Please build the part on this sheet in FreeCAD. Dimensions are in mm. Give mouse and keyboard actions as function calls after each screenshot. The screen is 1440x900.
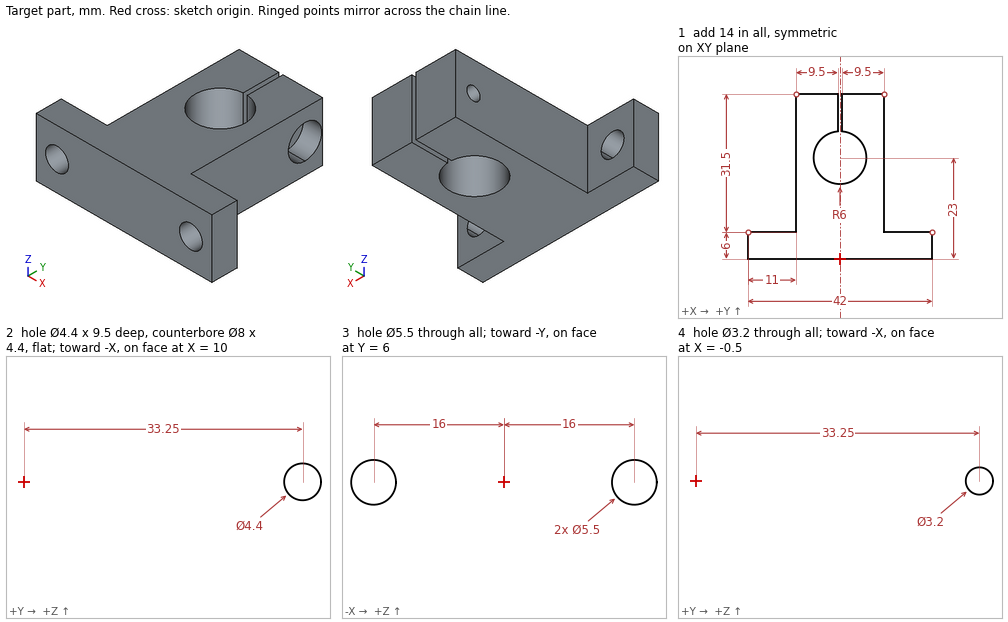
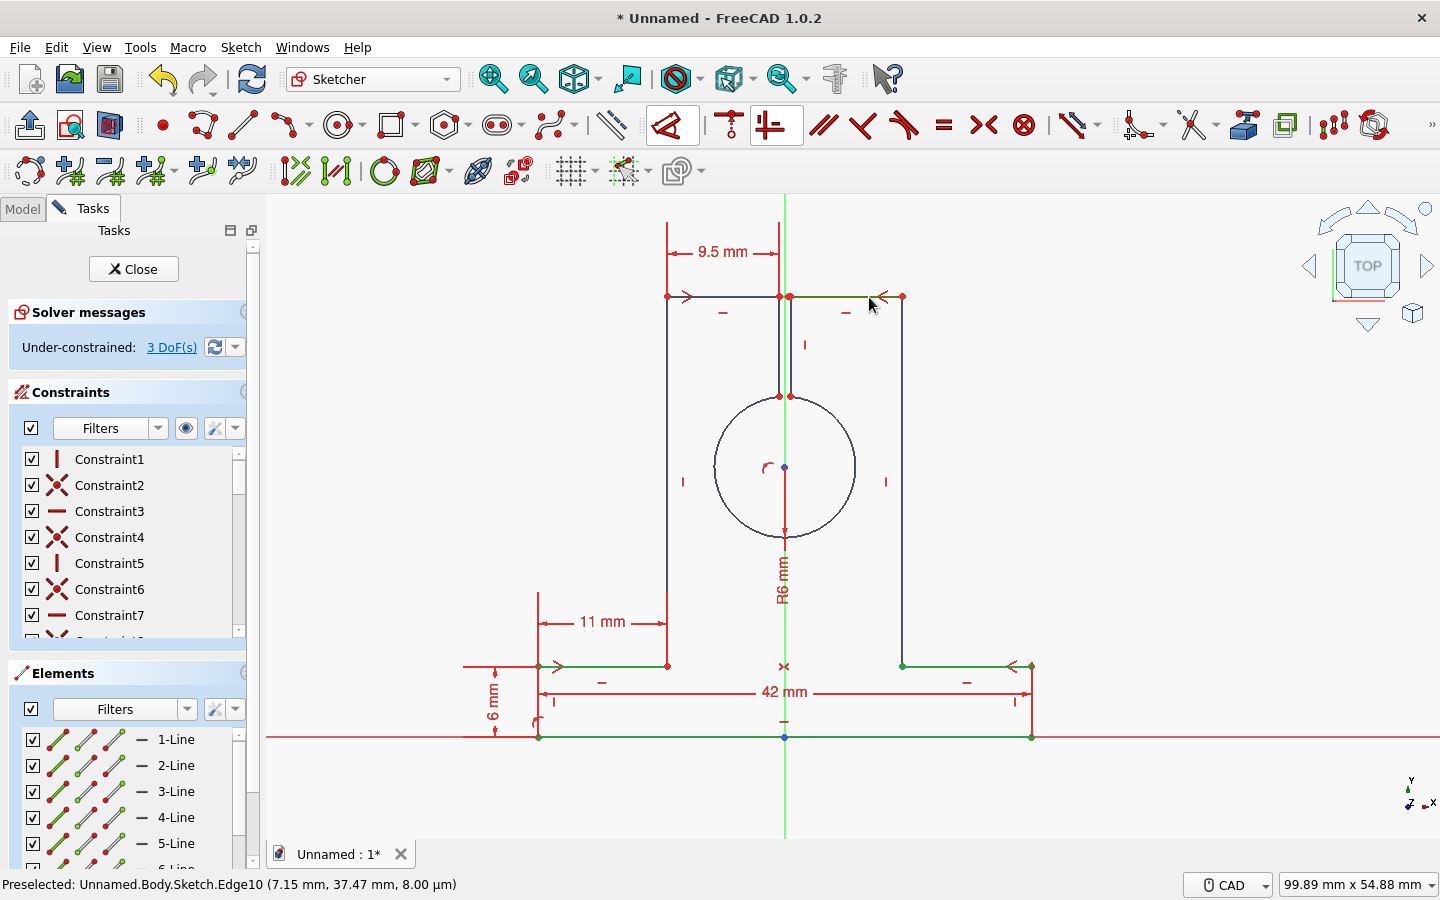
click(694, 126)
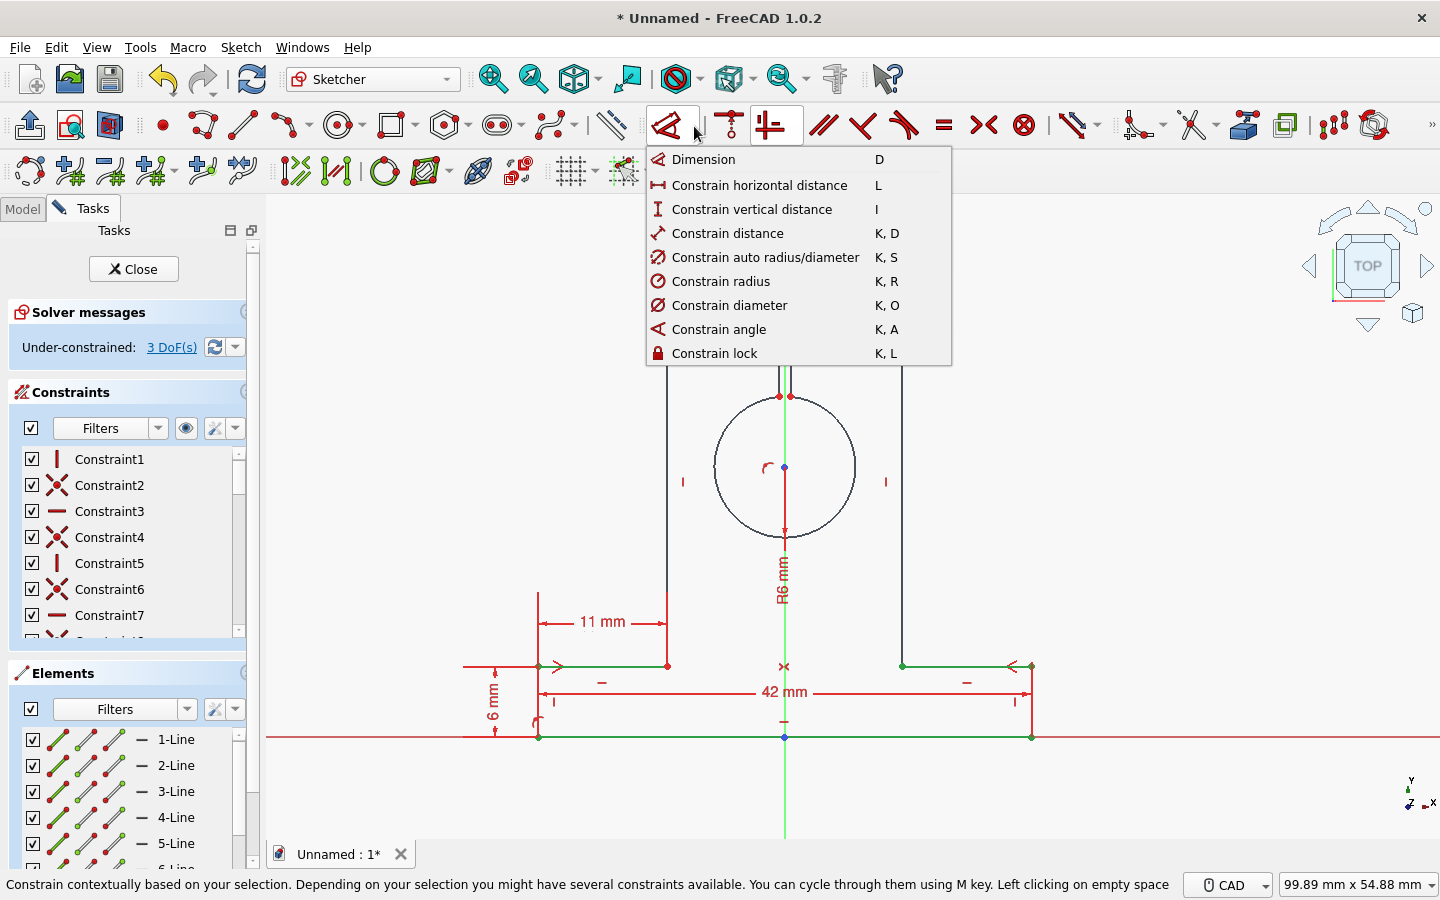
click(799, 185)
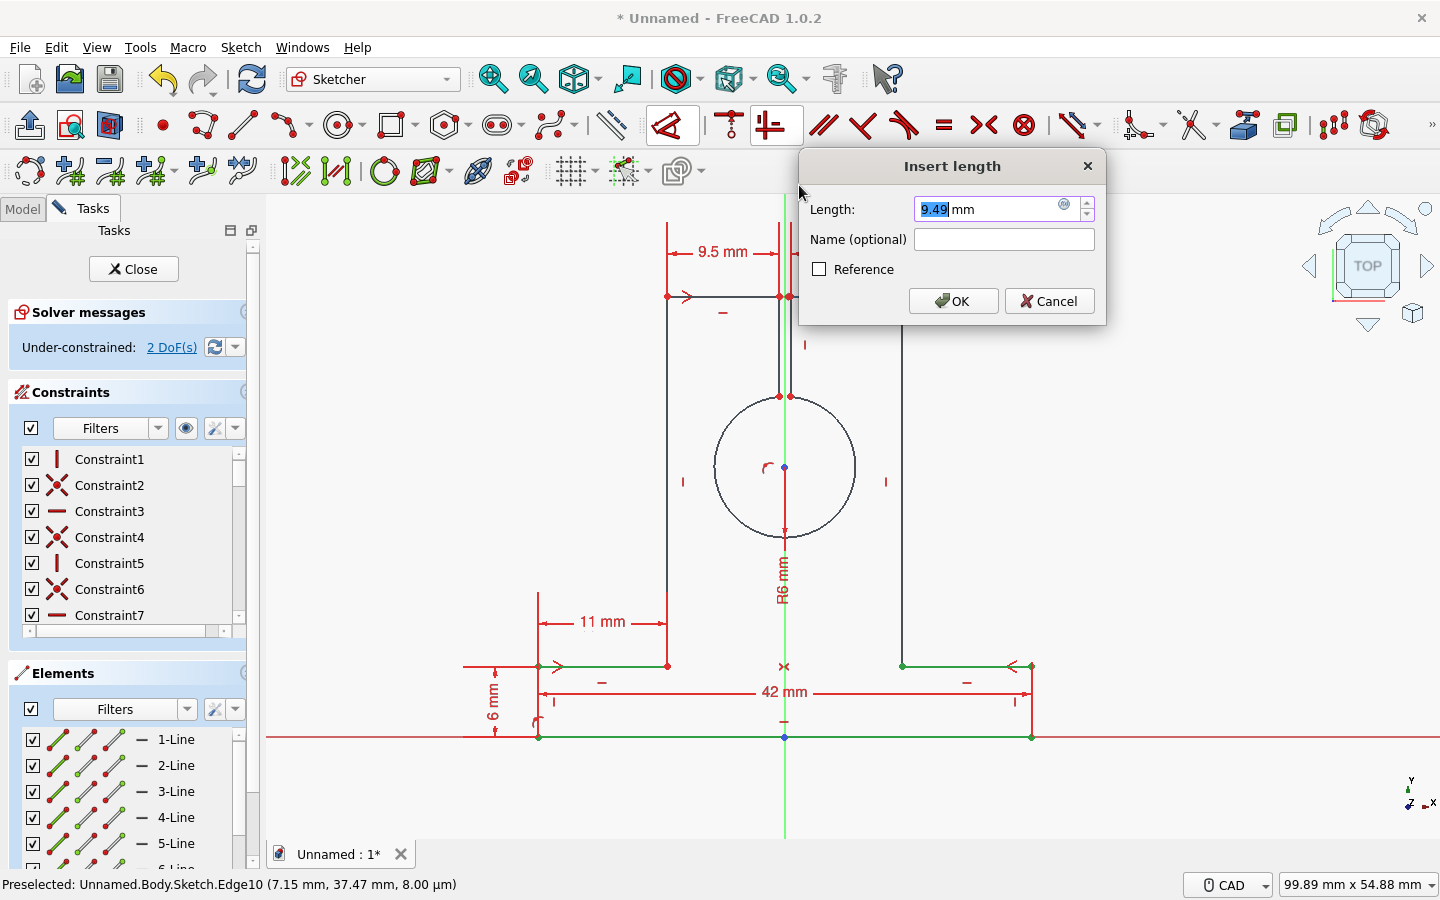
text(9.5)
key(Return)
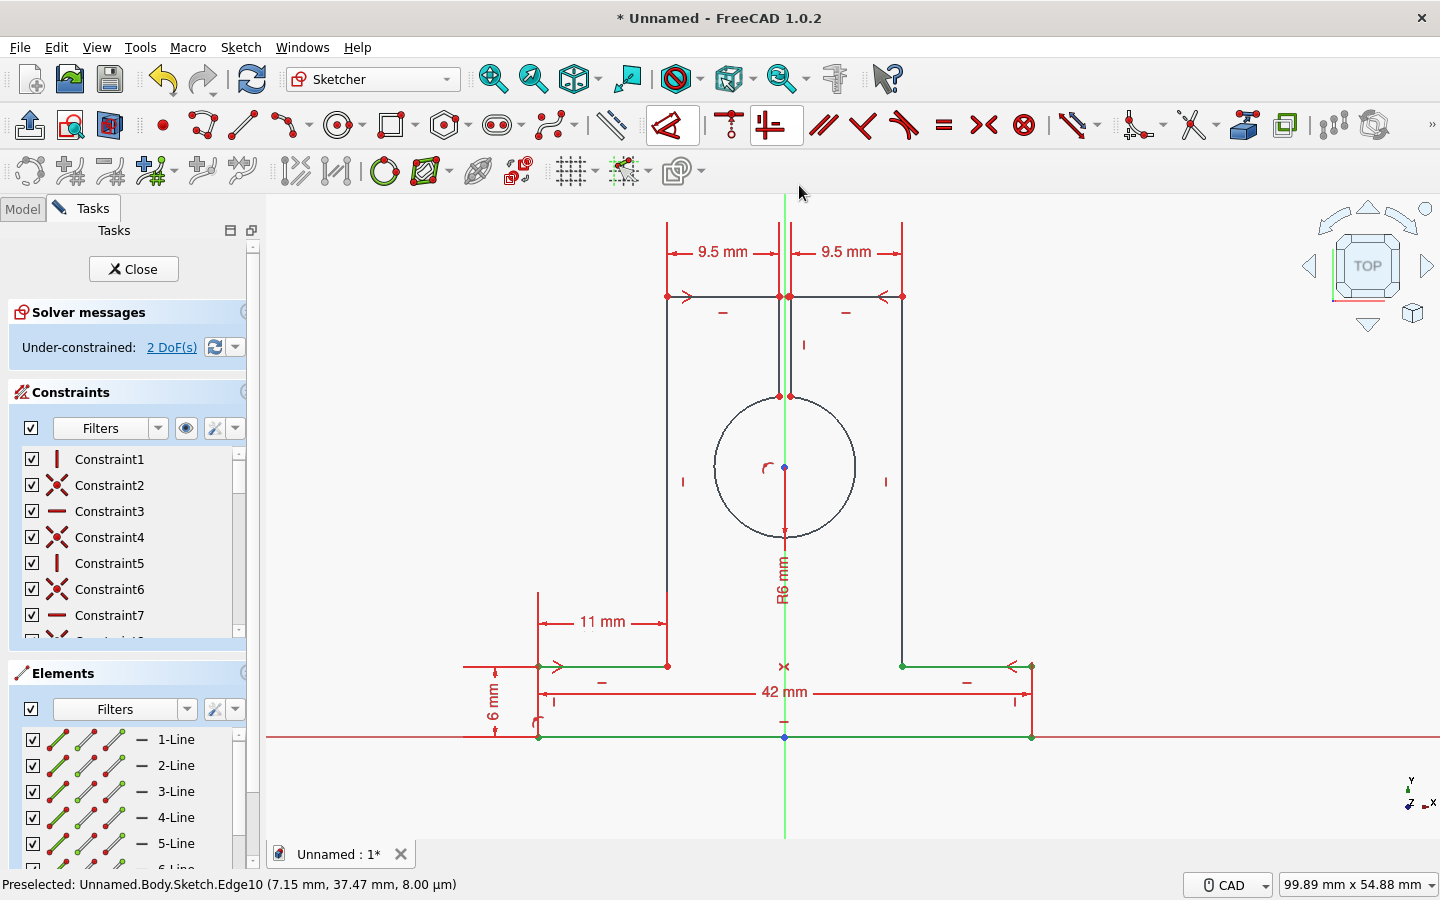
click(785, 467)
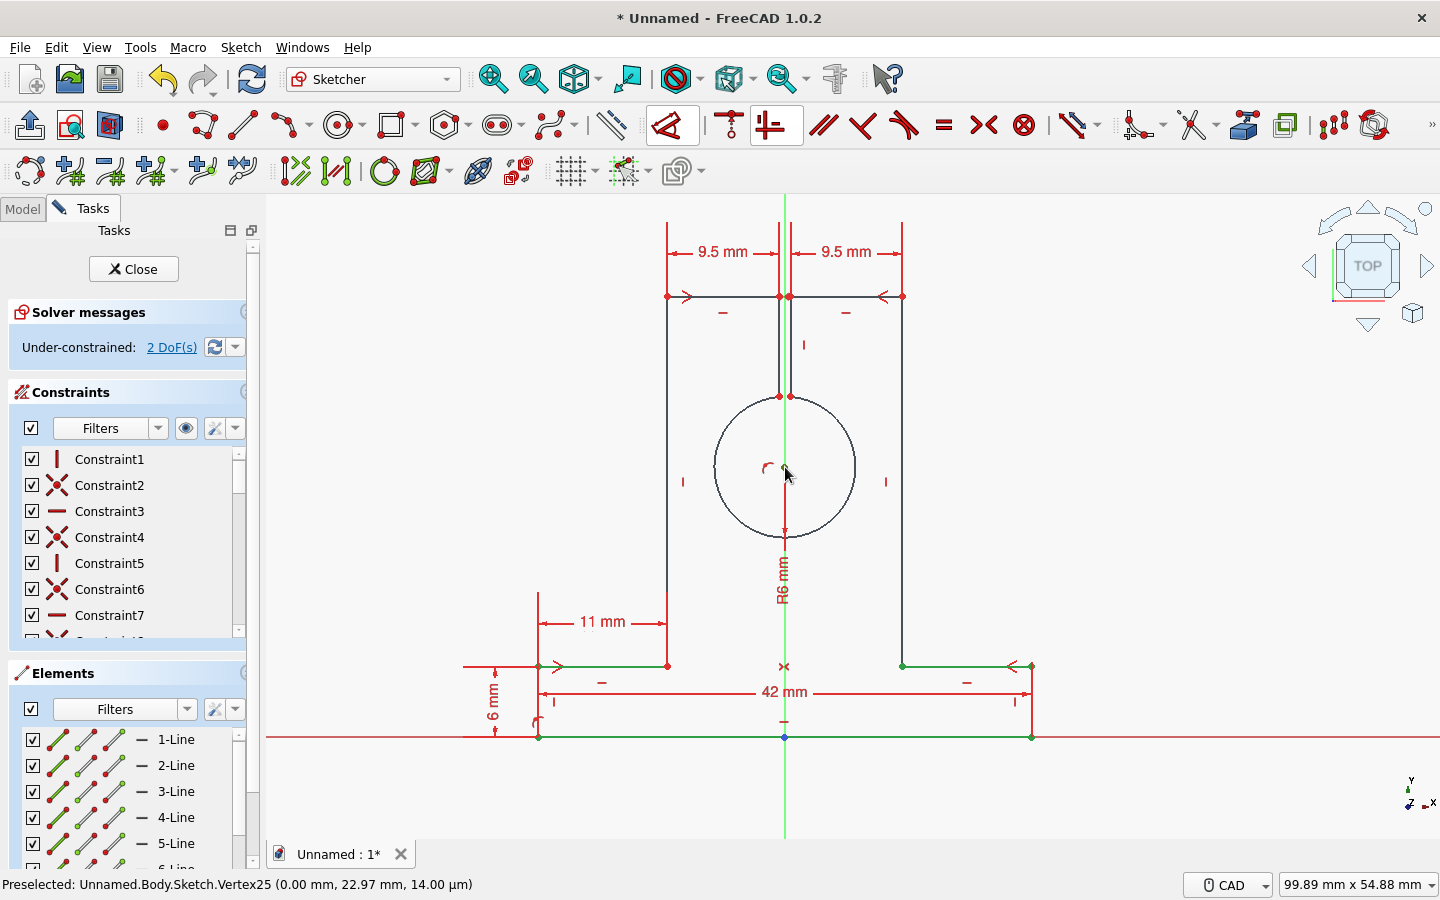
key(i)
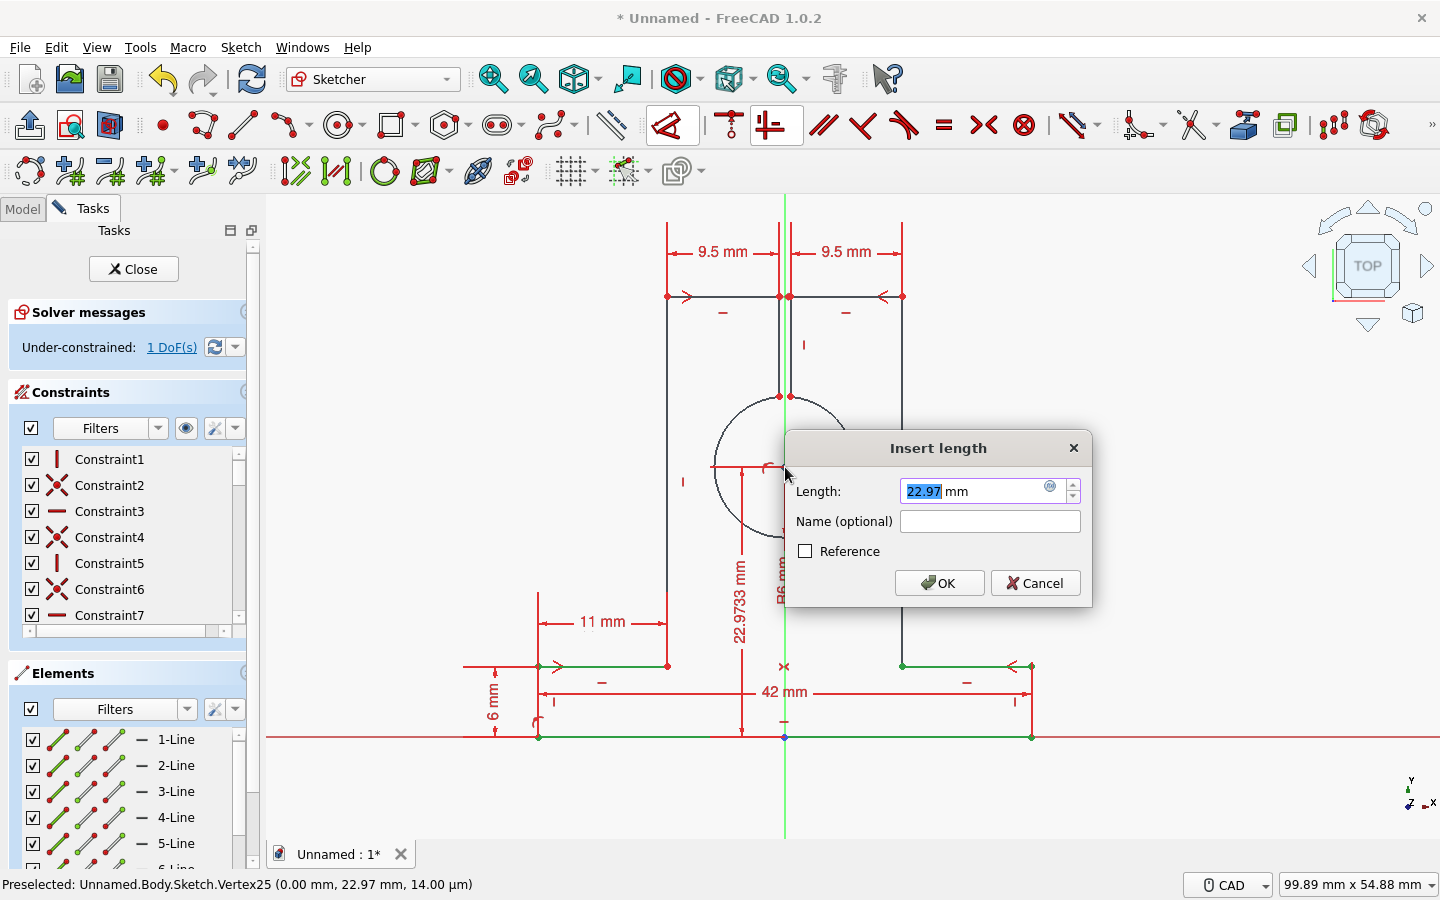
text(23)
key(Return)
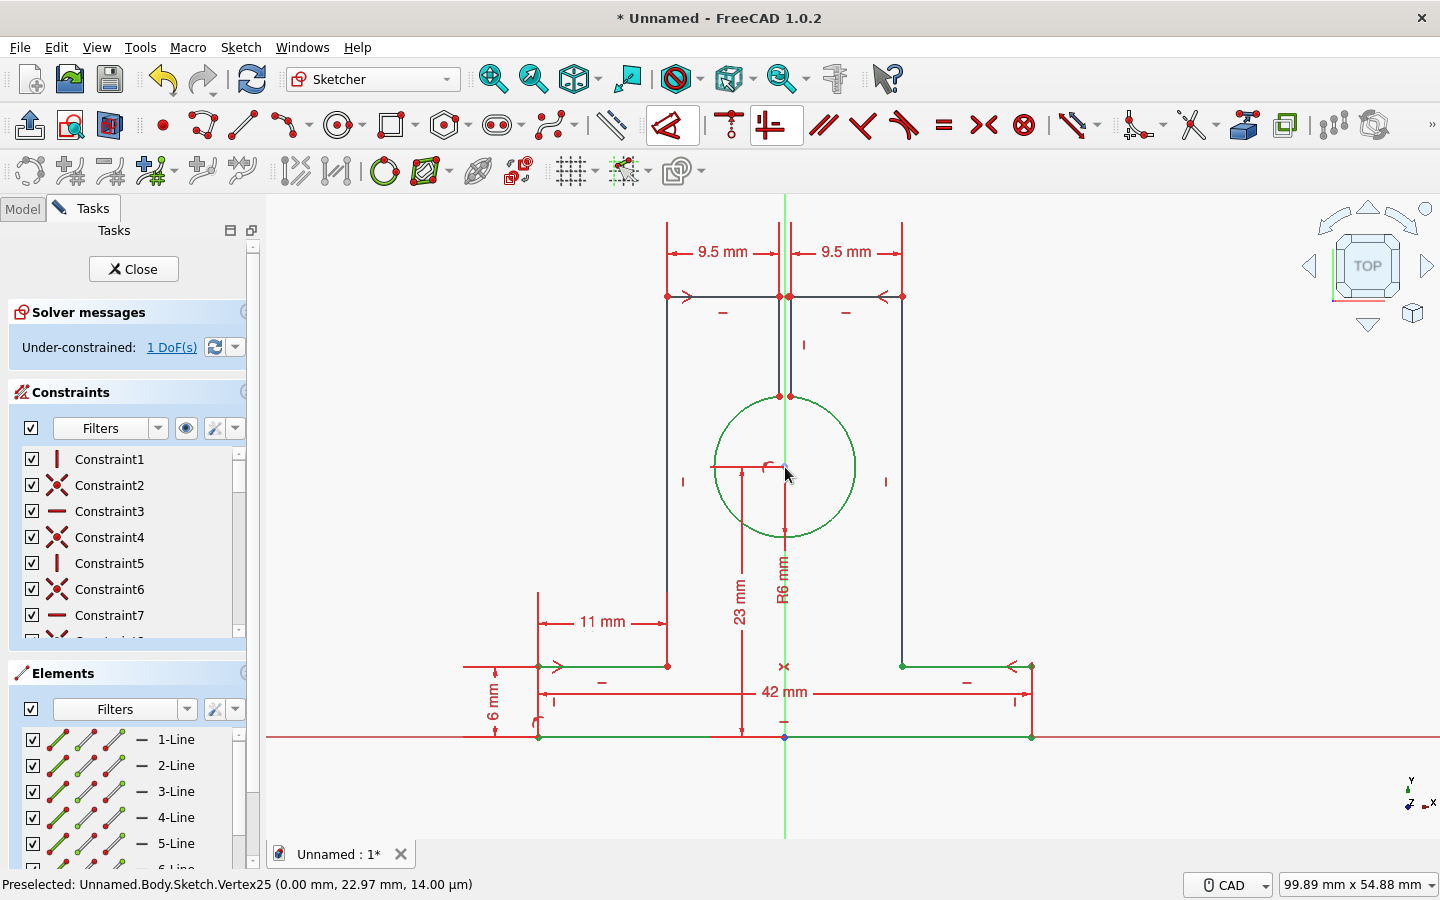
click(667, 408)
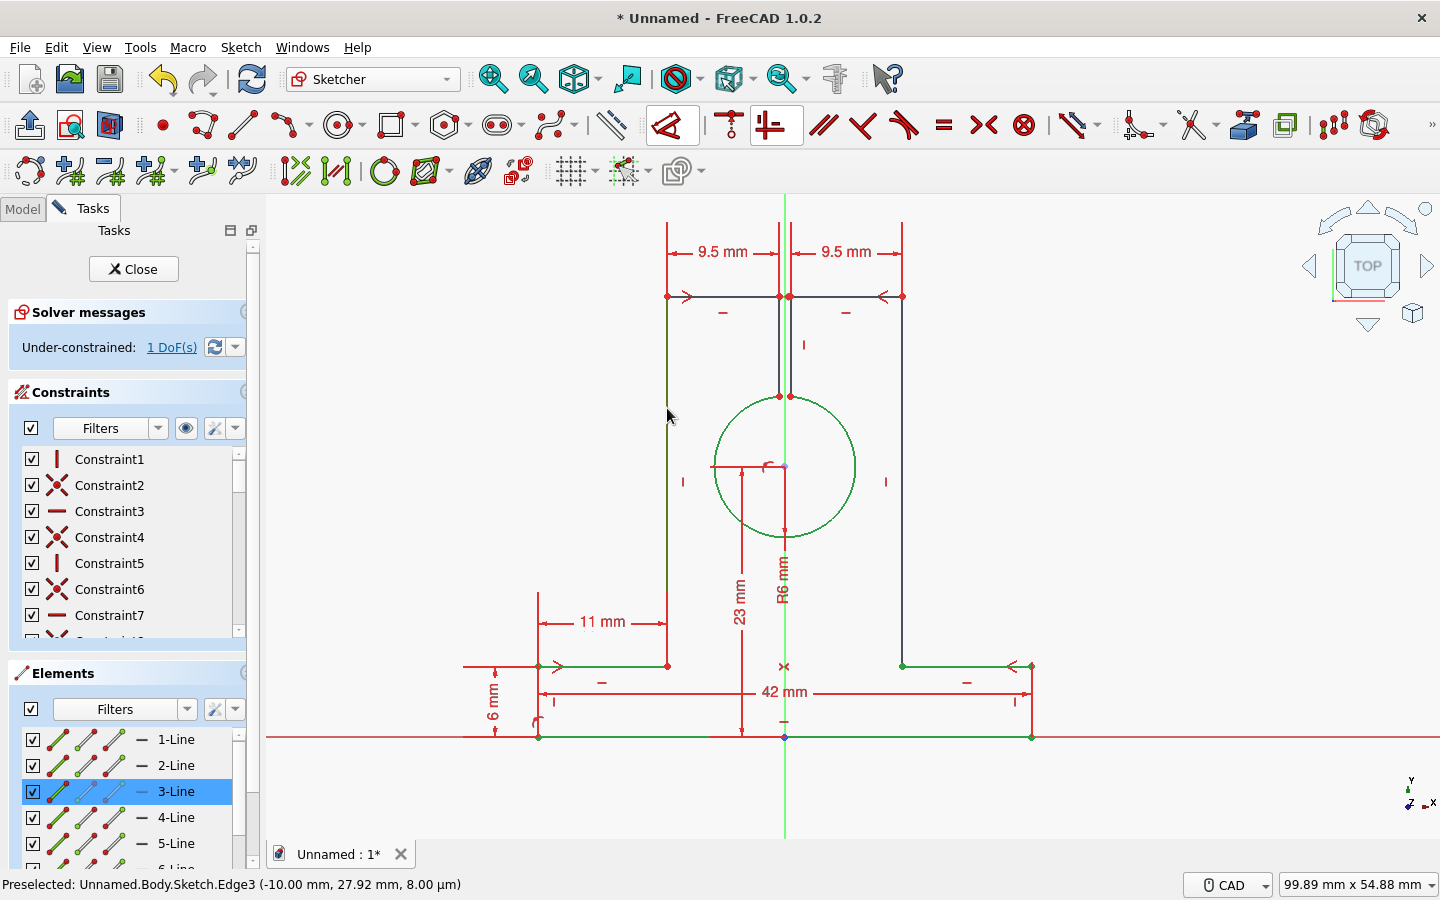
key(i)